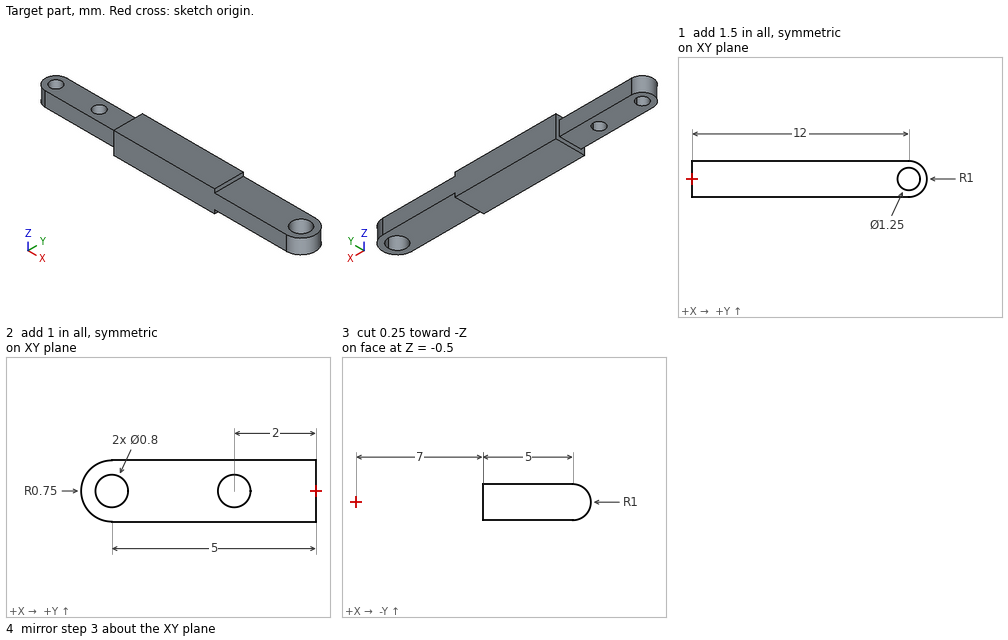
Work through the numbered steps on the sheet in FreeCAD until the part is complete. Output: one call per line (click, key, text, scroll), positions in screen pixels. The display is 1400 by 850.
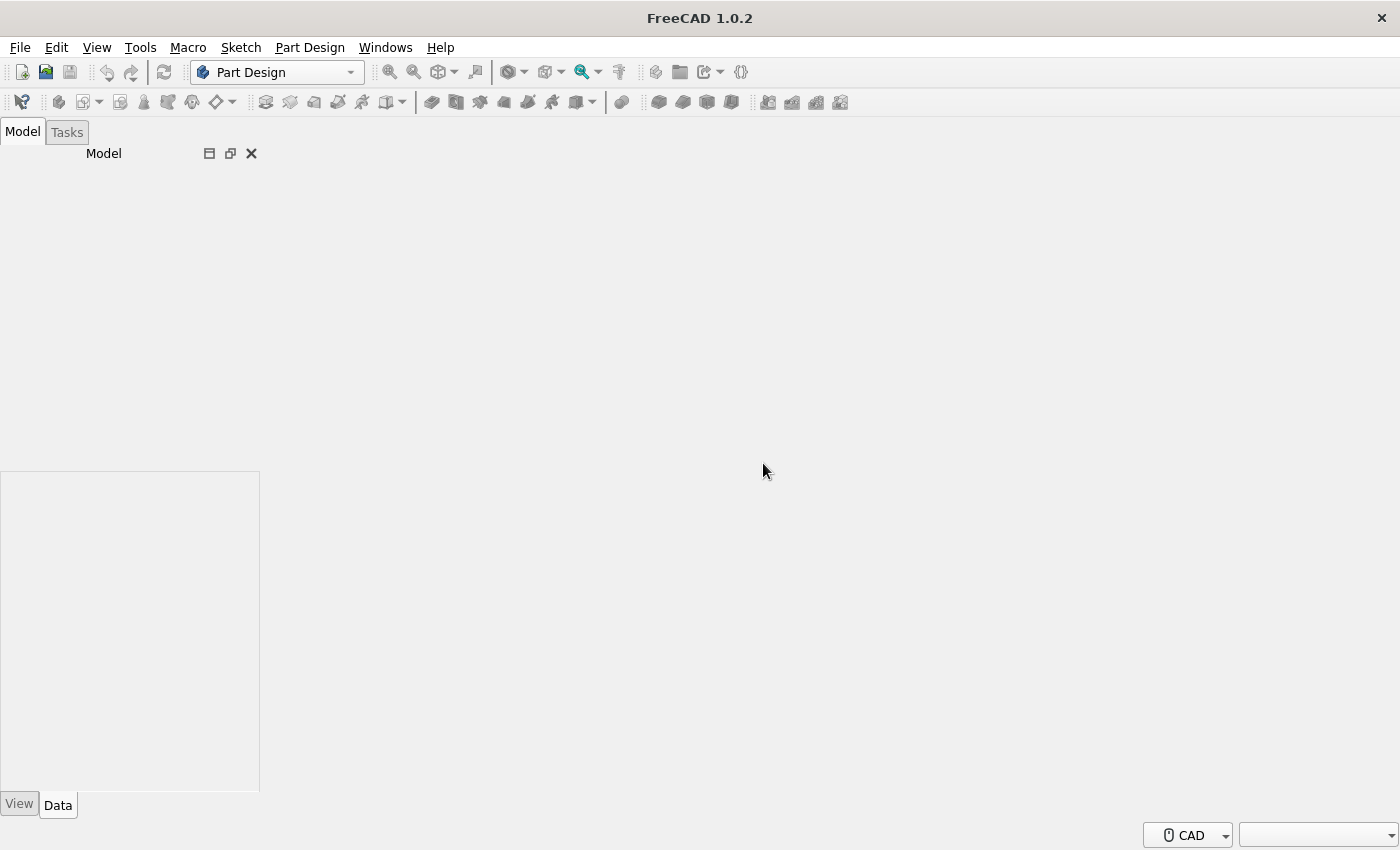
key(ctrl+n)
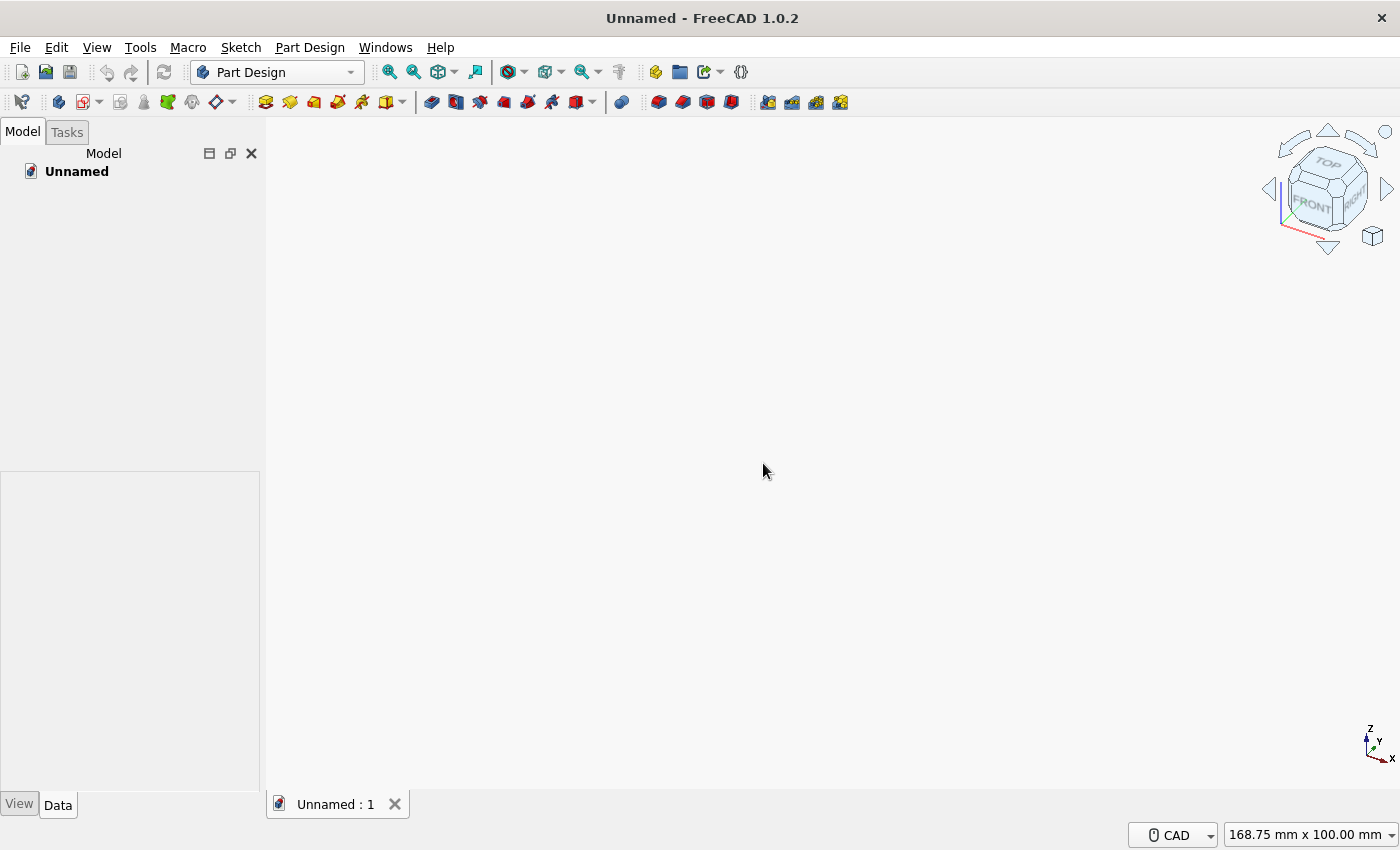
click(84, 102)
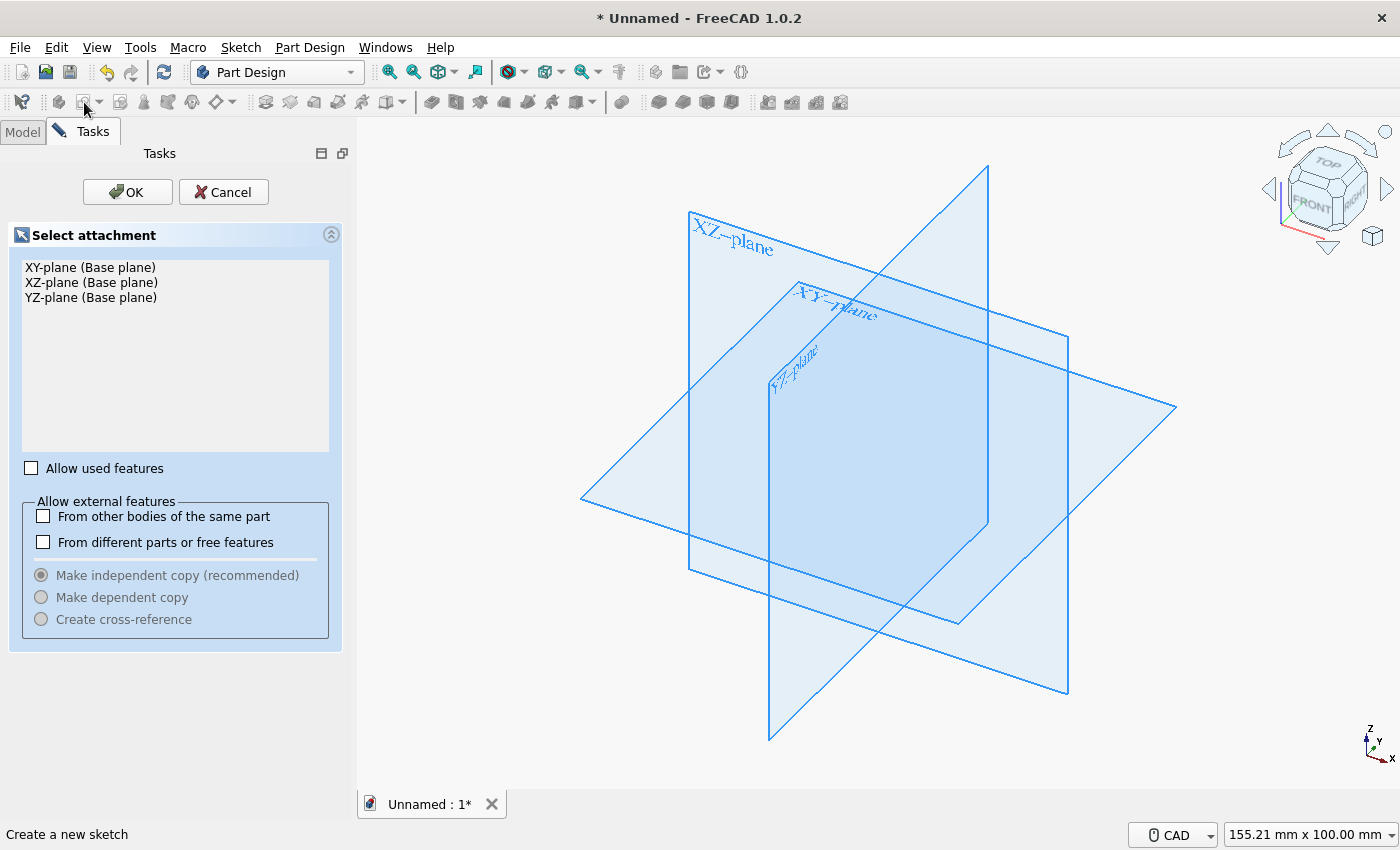
click(82, 268)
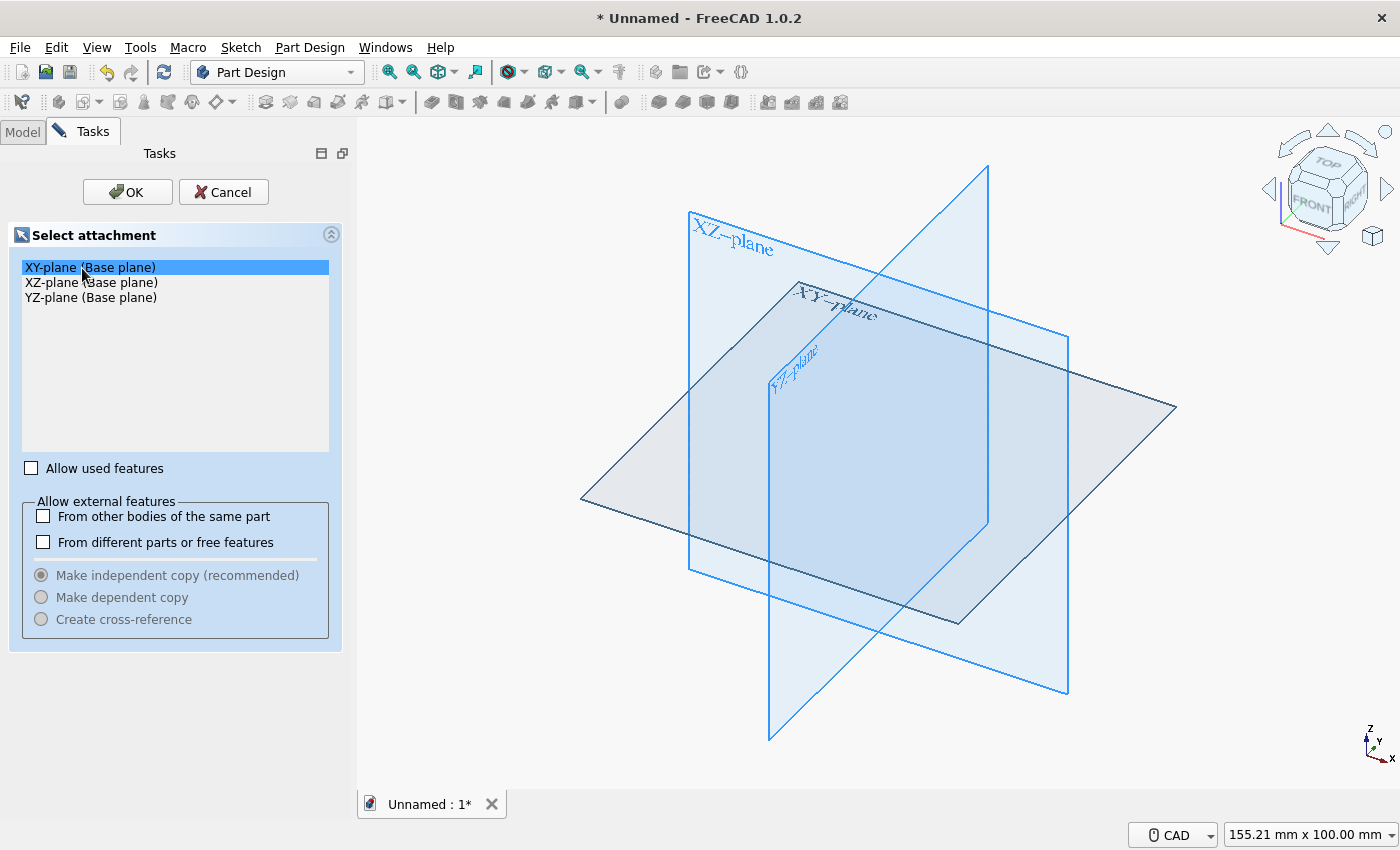
click(128, 192)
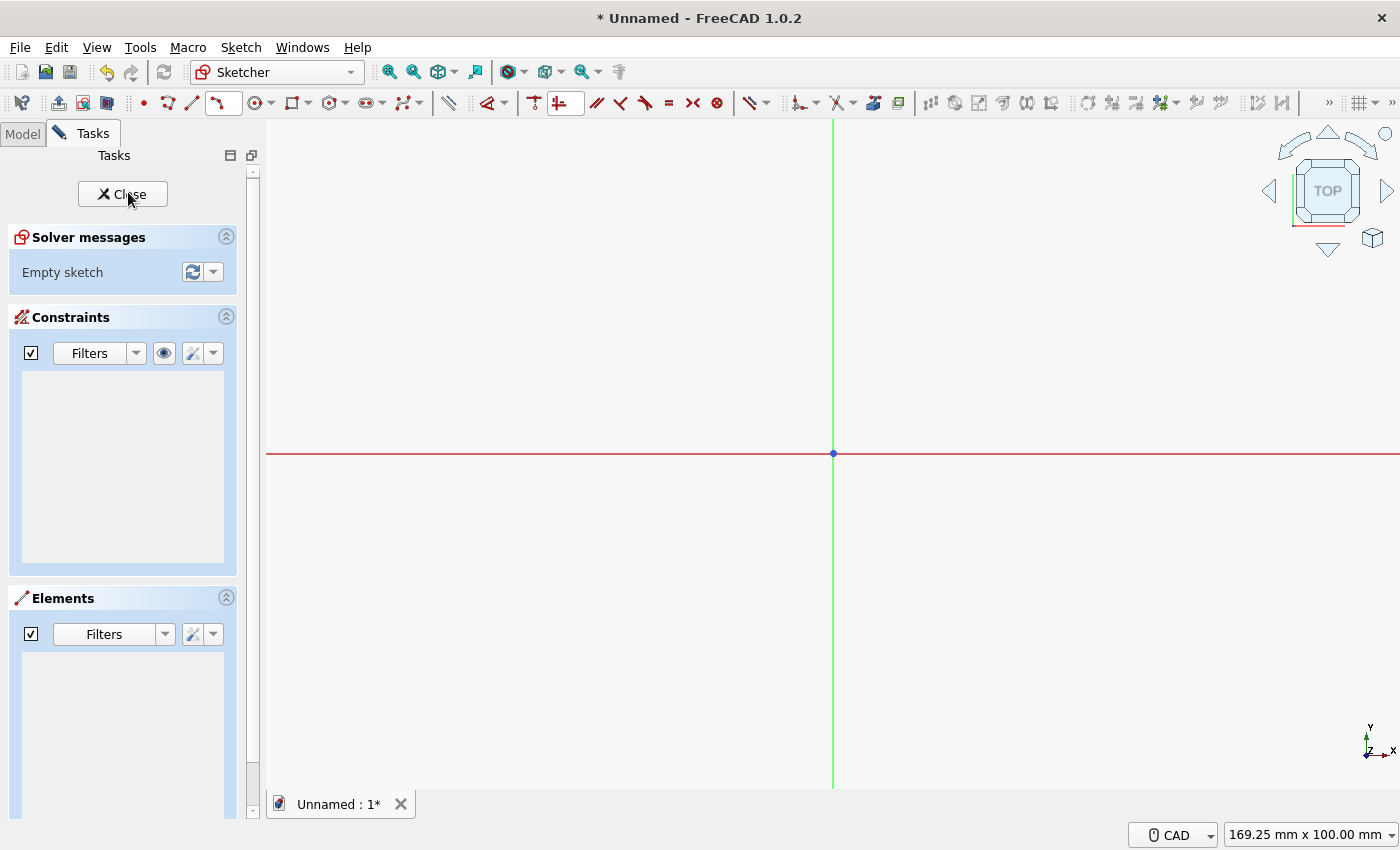
scroll(894, 454, up, 10)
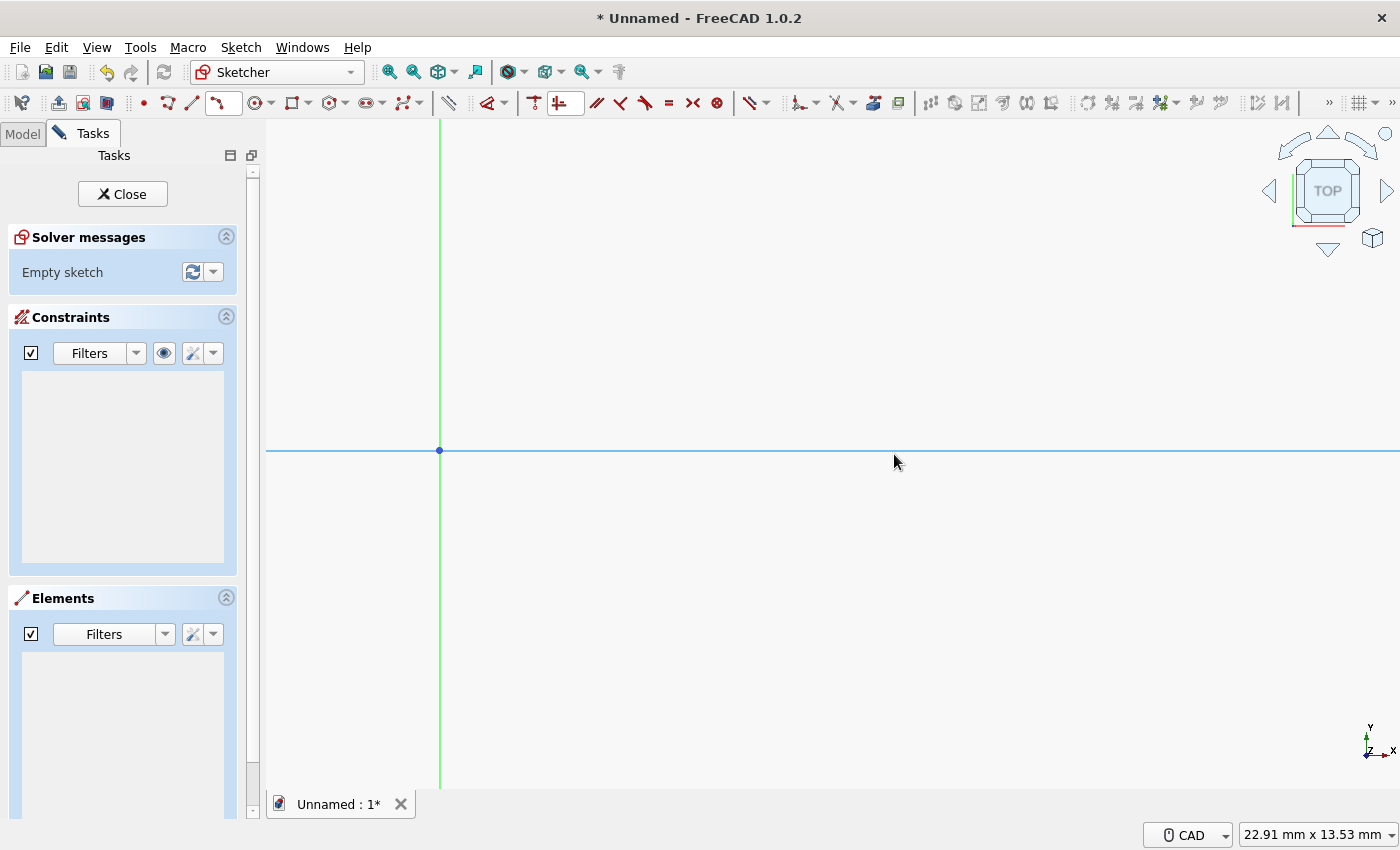
click(168, 104)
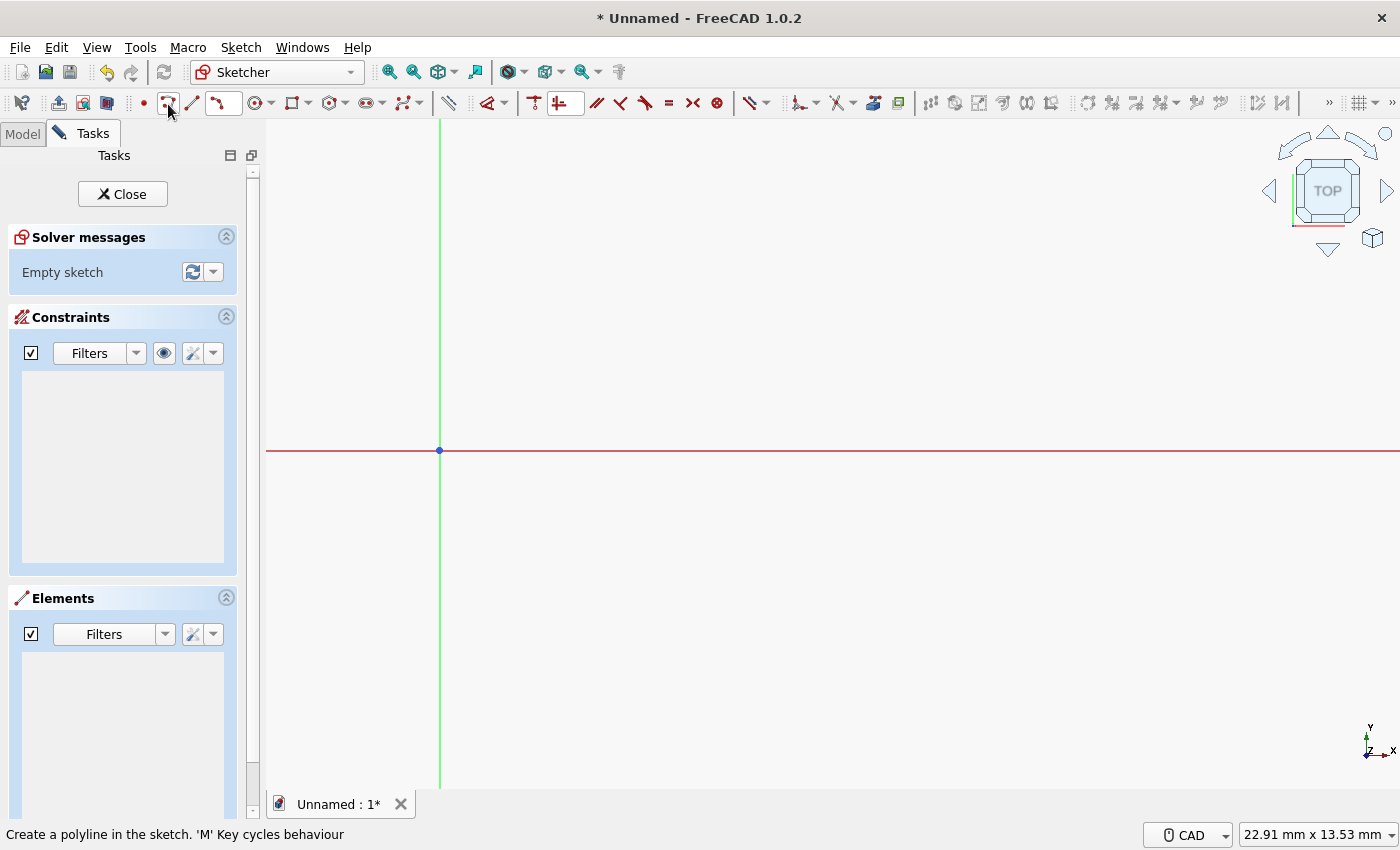
click(1034, 401)
click(440, 401)
click(449, 500)
click(1034, 500)
right_click(1034, 500)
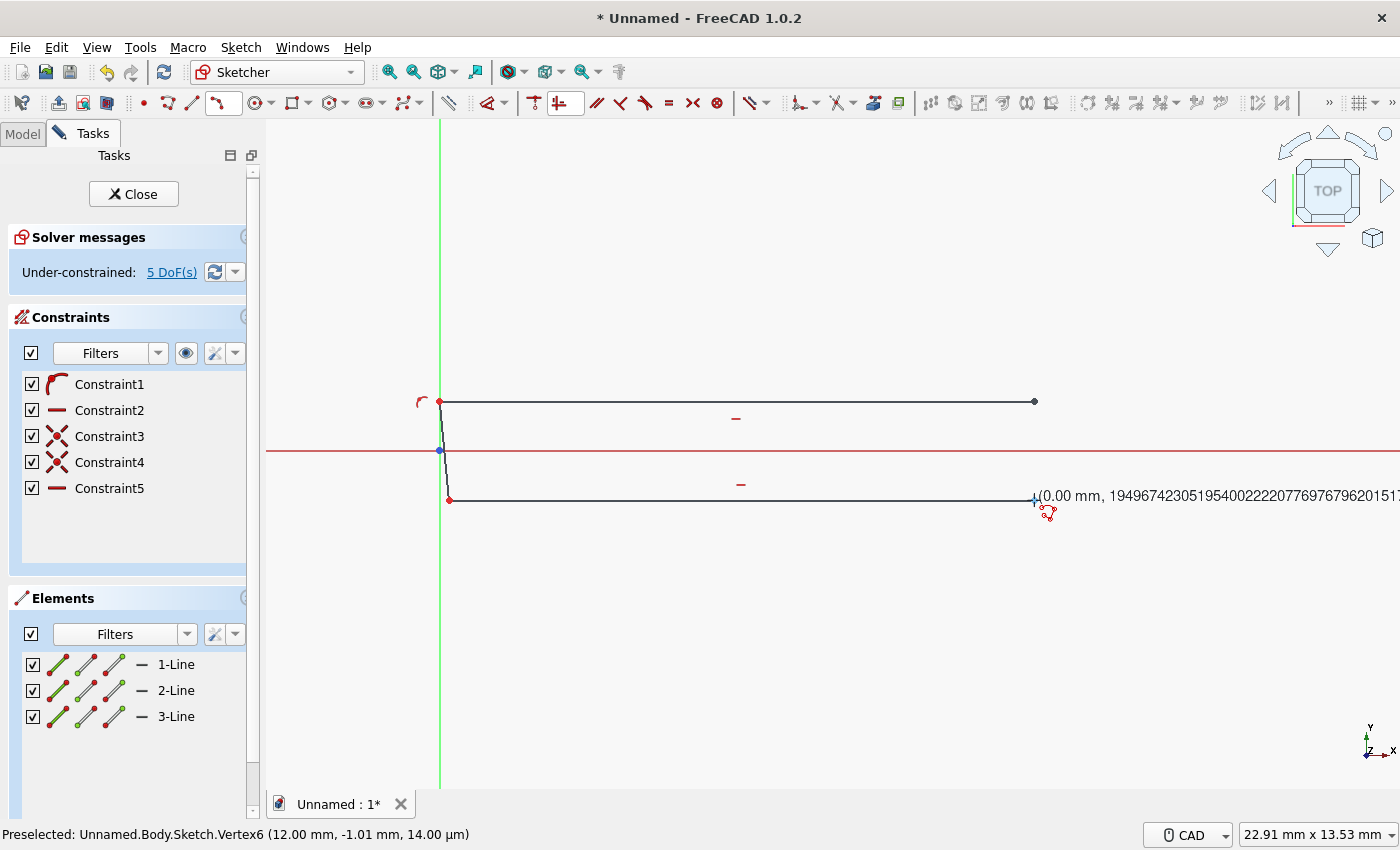
click(218, 104)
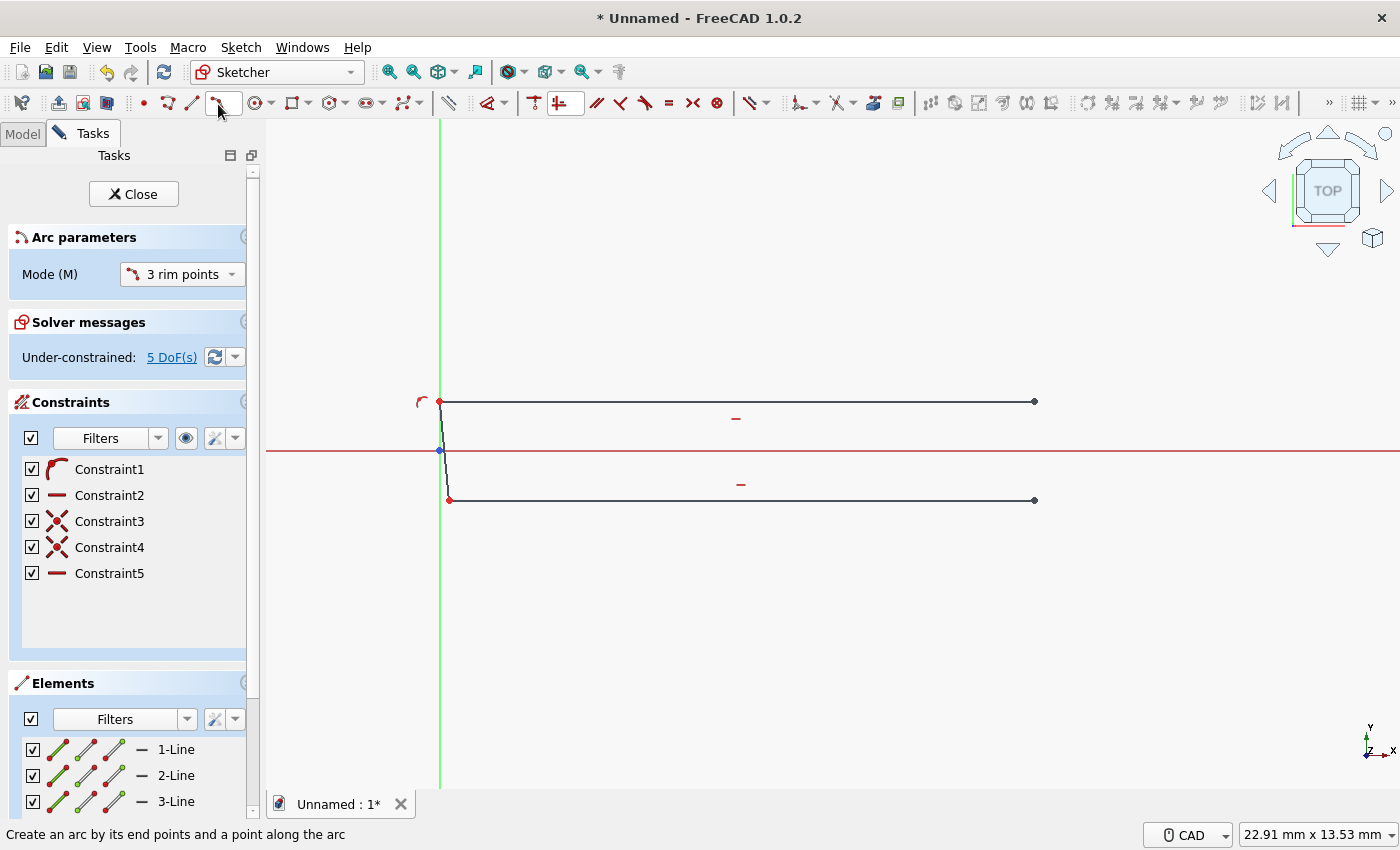
click(1034, 501)
click(1034, 402)
click(1081, 466)